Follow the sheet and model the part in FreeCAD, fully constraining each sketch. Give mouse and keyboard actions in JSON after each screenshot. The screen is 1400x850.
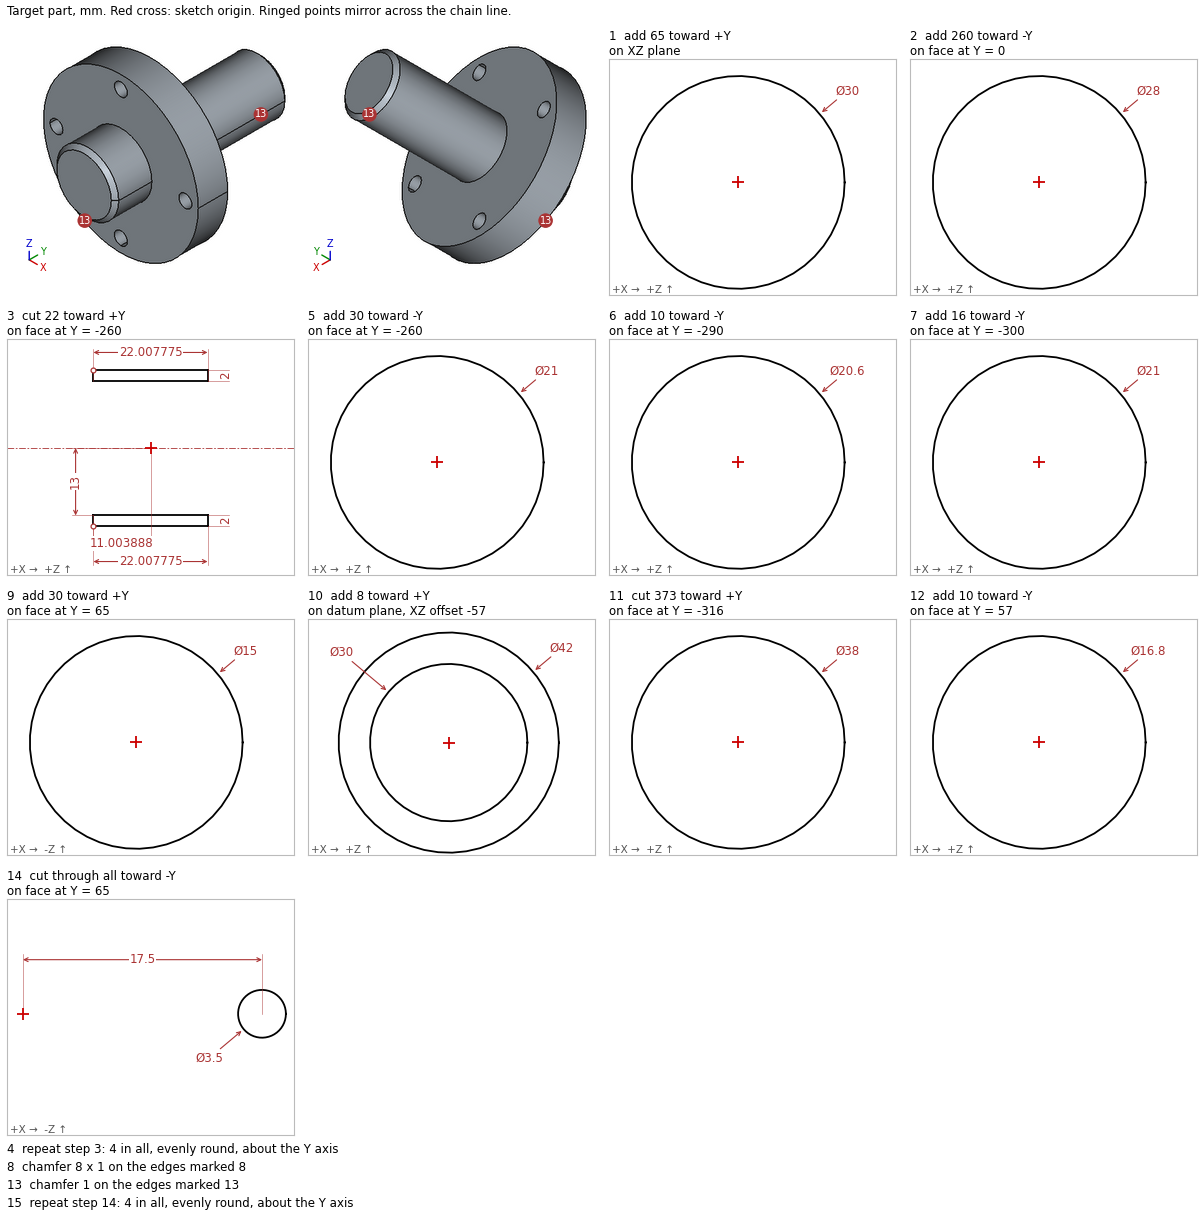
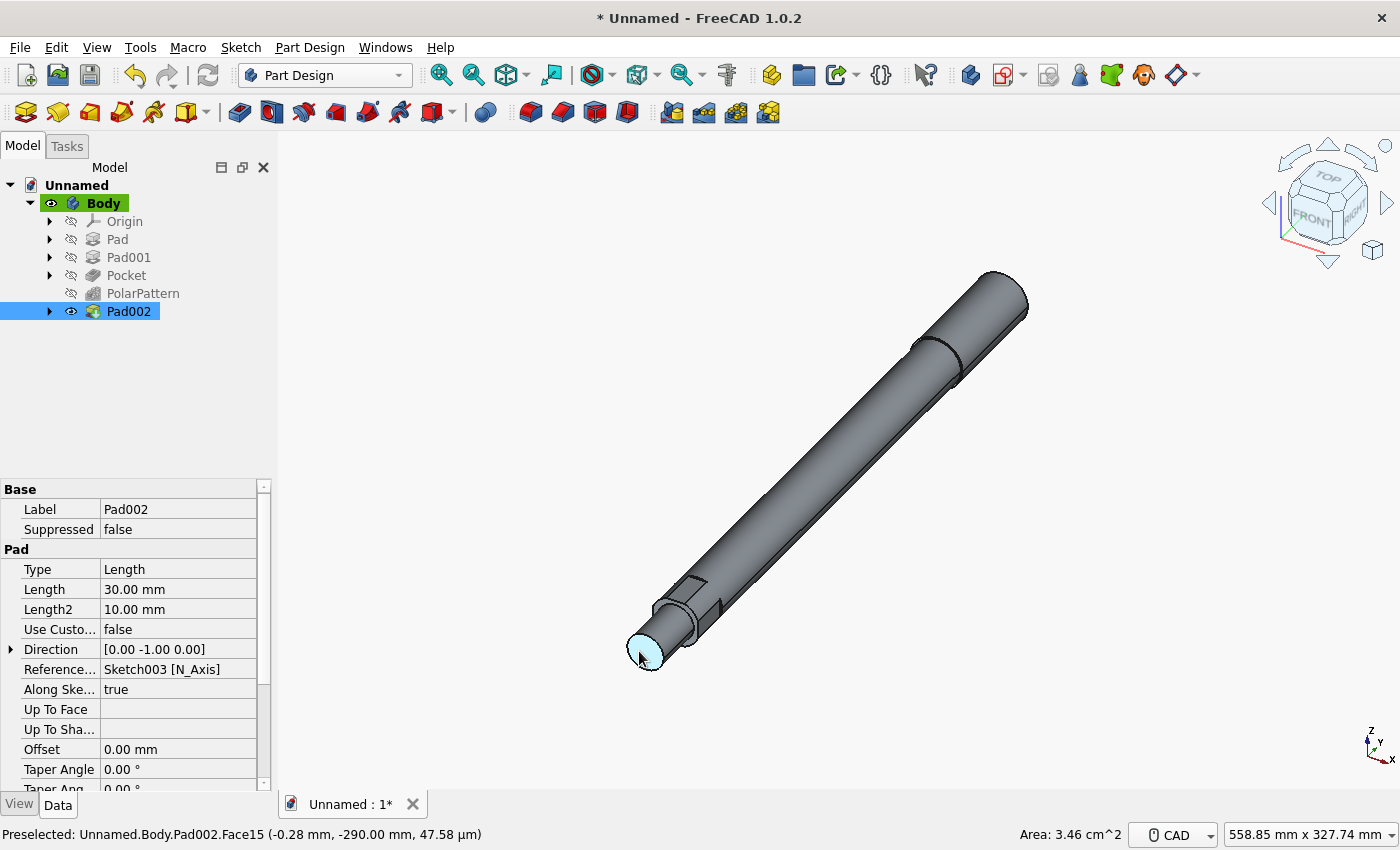
{"action": "left_click", "coordinate": [1004, 76]}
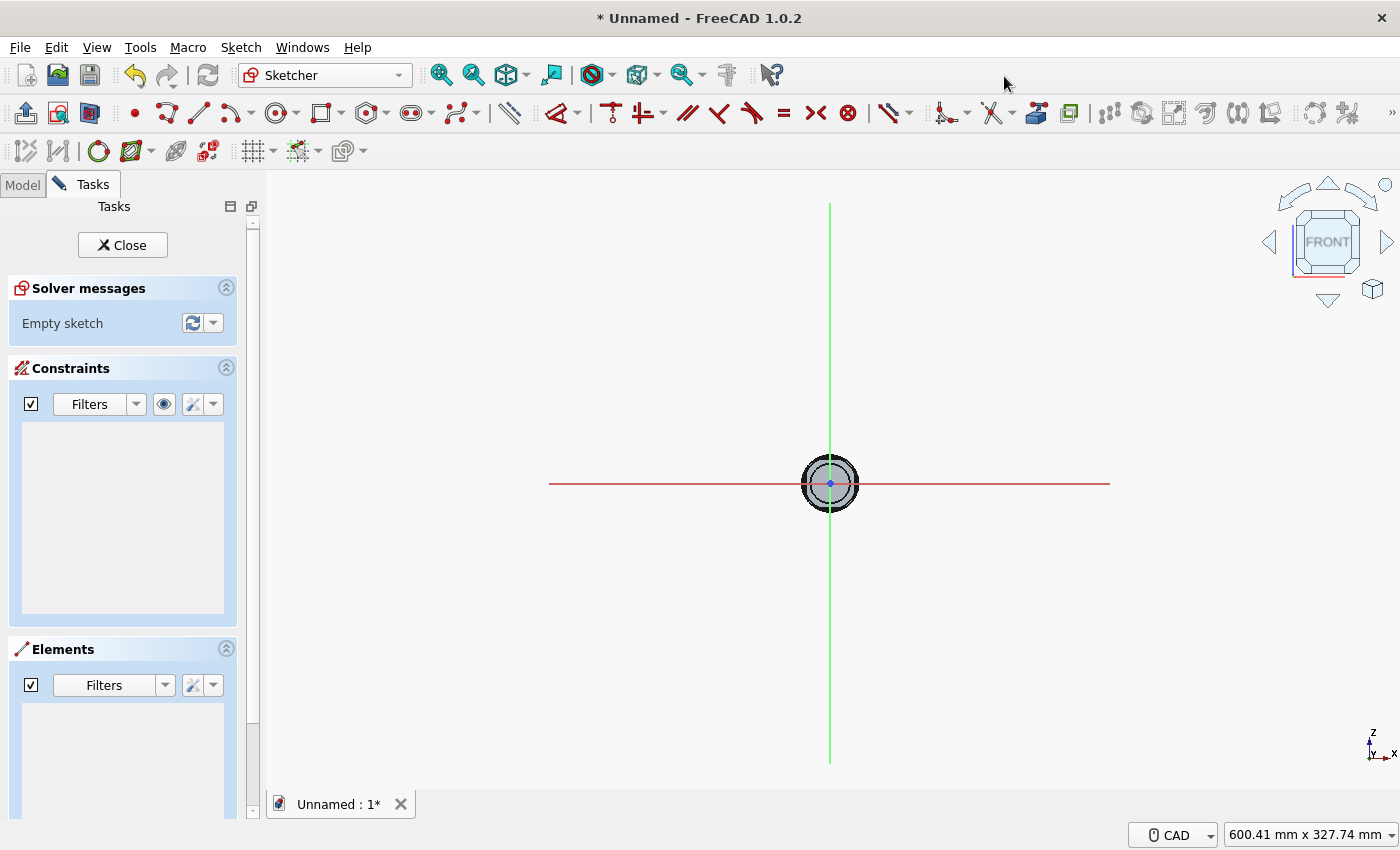
{"action": "scroll", "coordinate": [837, 484], "scroll_direction": "up", "scroll_amount": 12}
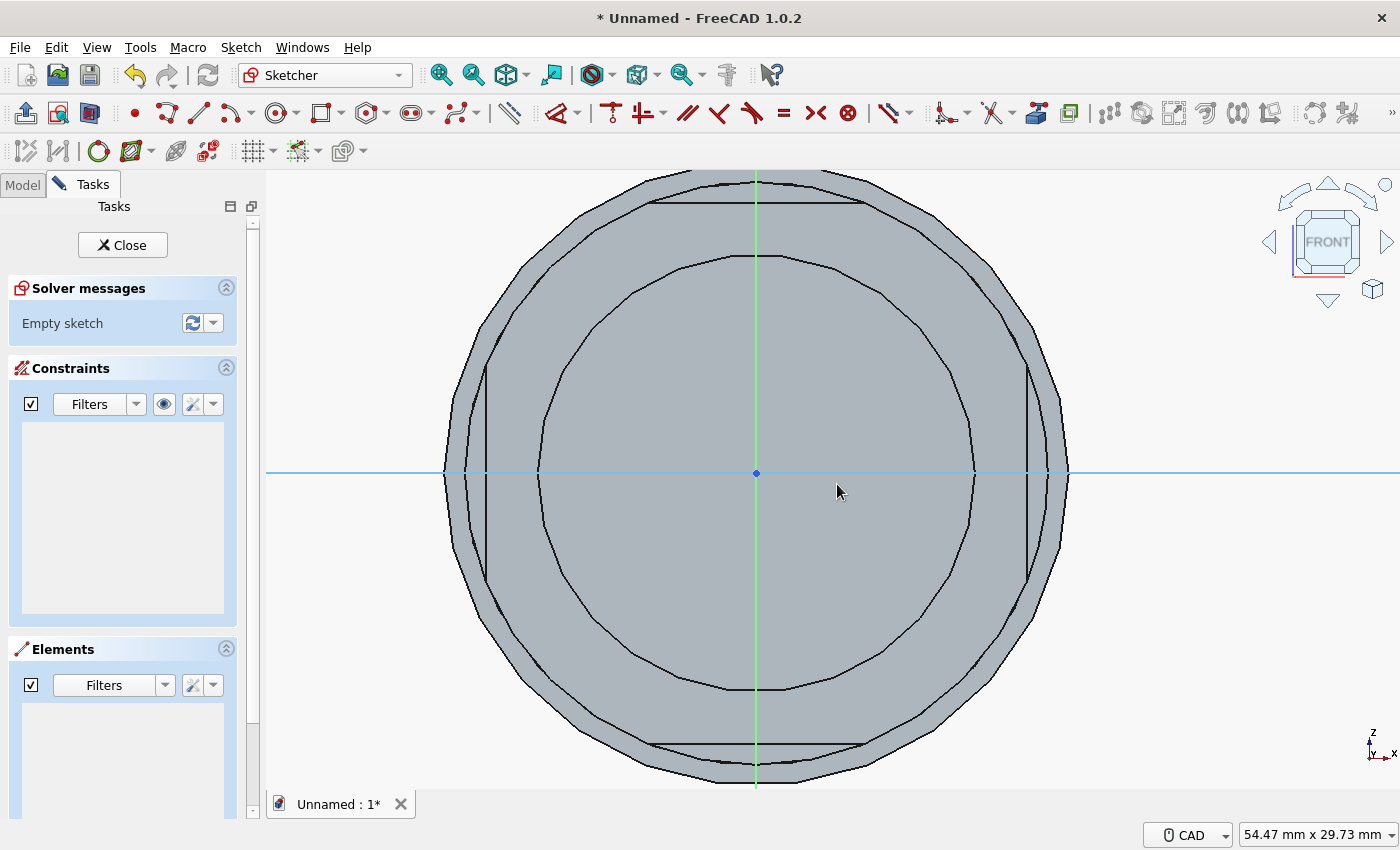
{"action": "left_click", "coordinate": [276, 114]}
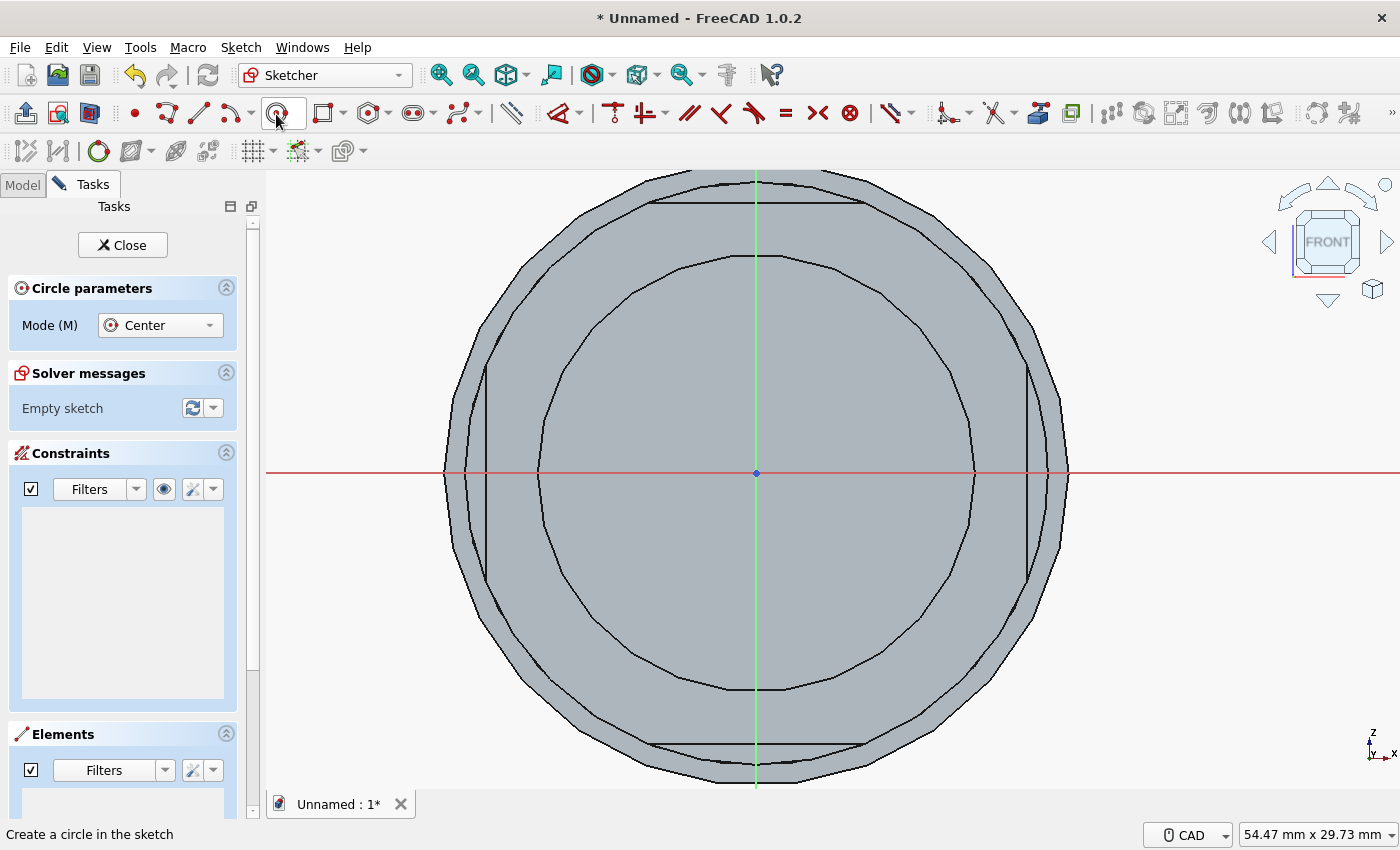
{"action": "left_click", "coordinate": [756, 473]}
{"action": "mouse_move", "coordinate": [908, 322]}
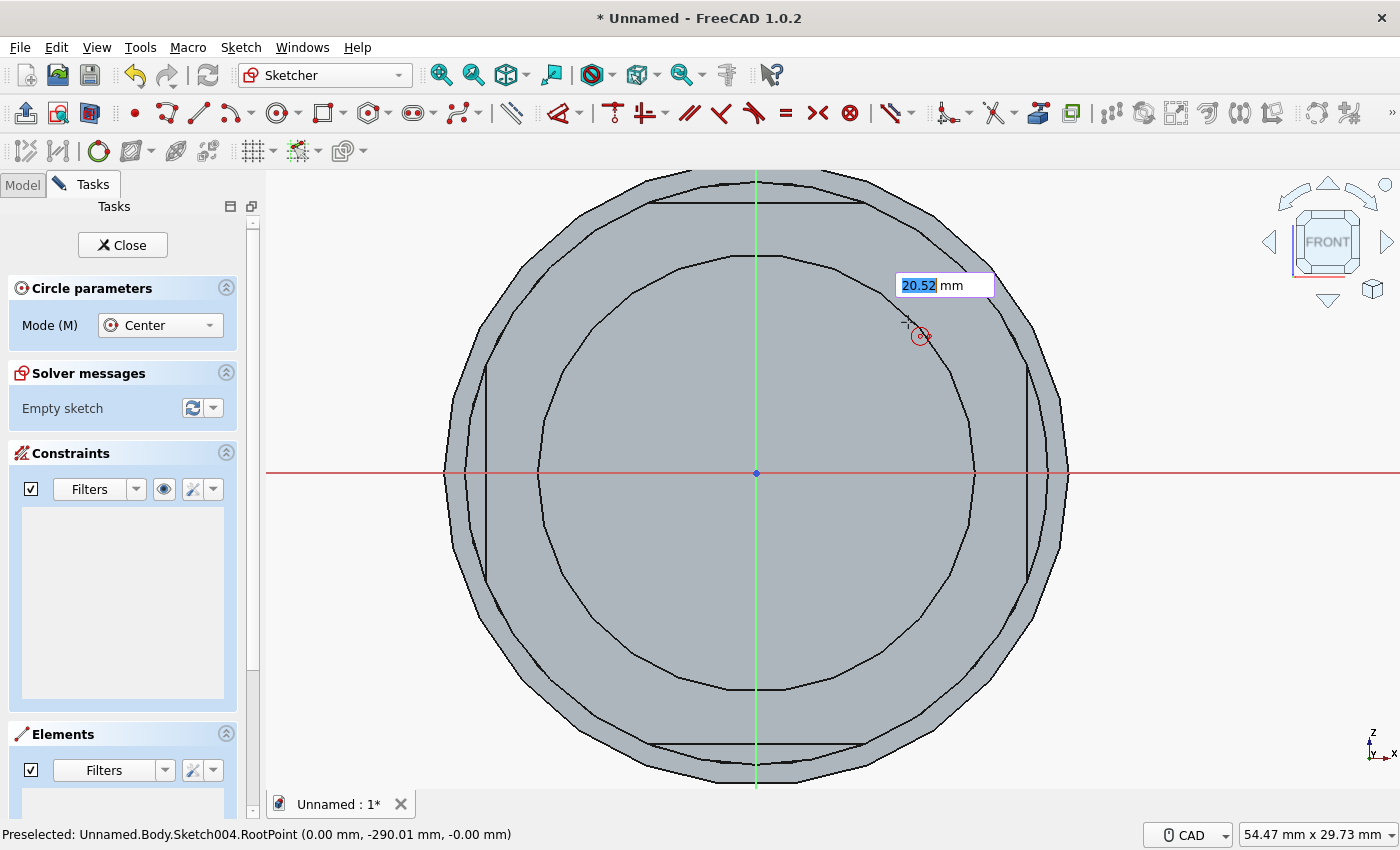
{"action": "type", "text": "20.6"}
{"action": "key", "text": "Return"}
{"action": "key", "text": "Escape"}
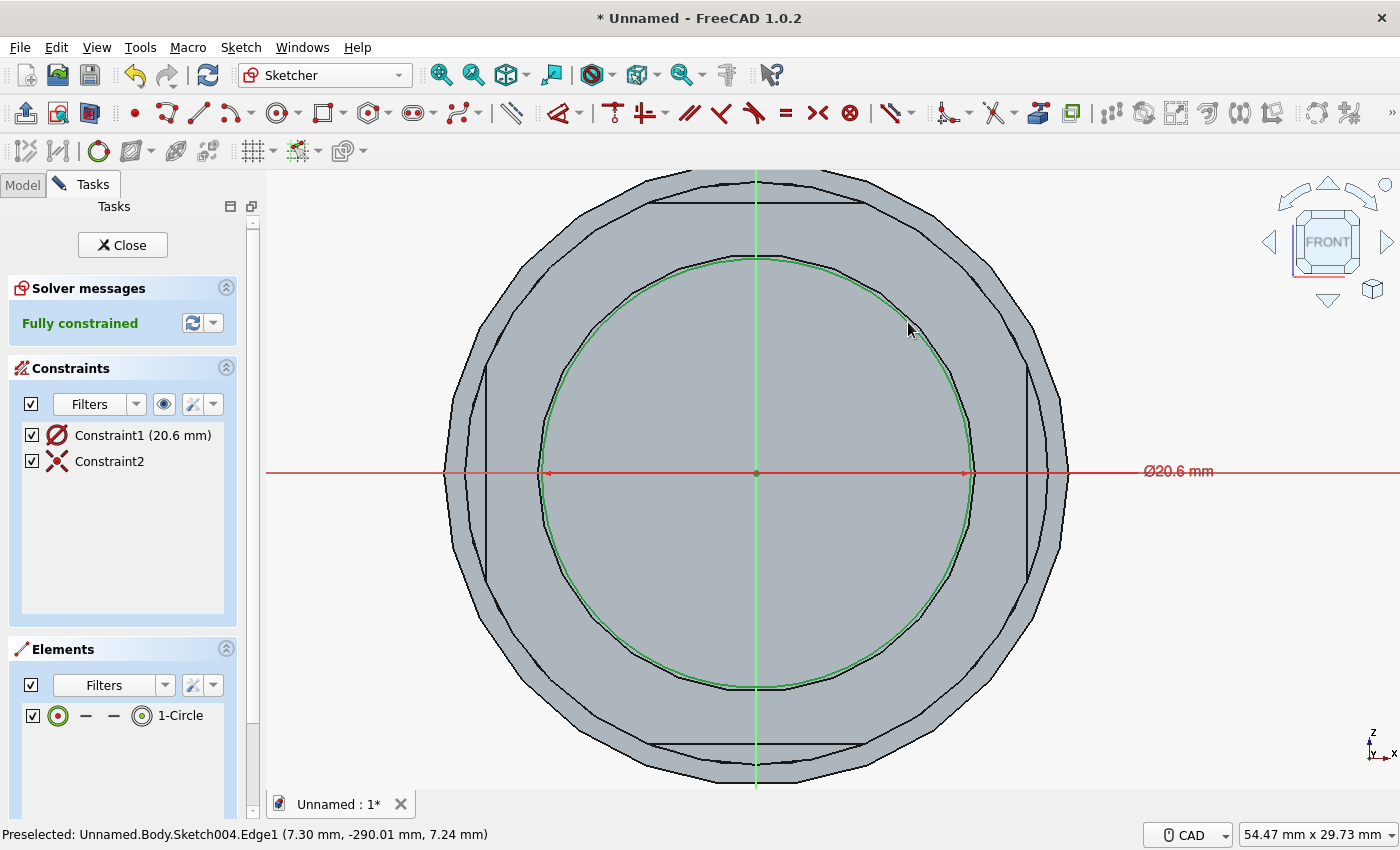
{"action": "left_click", "coordinate": [123, 245]}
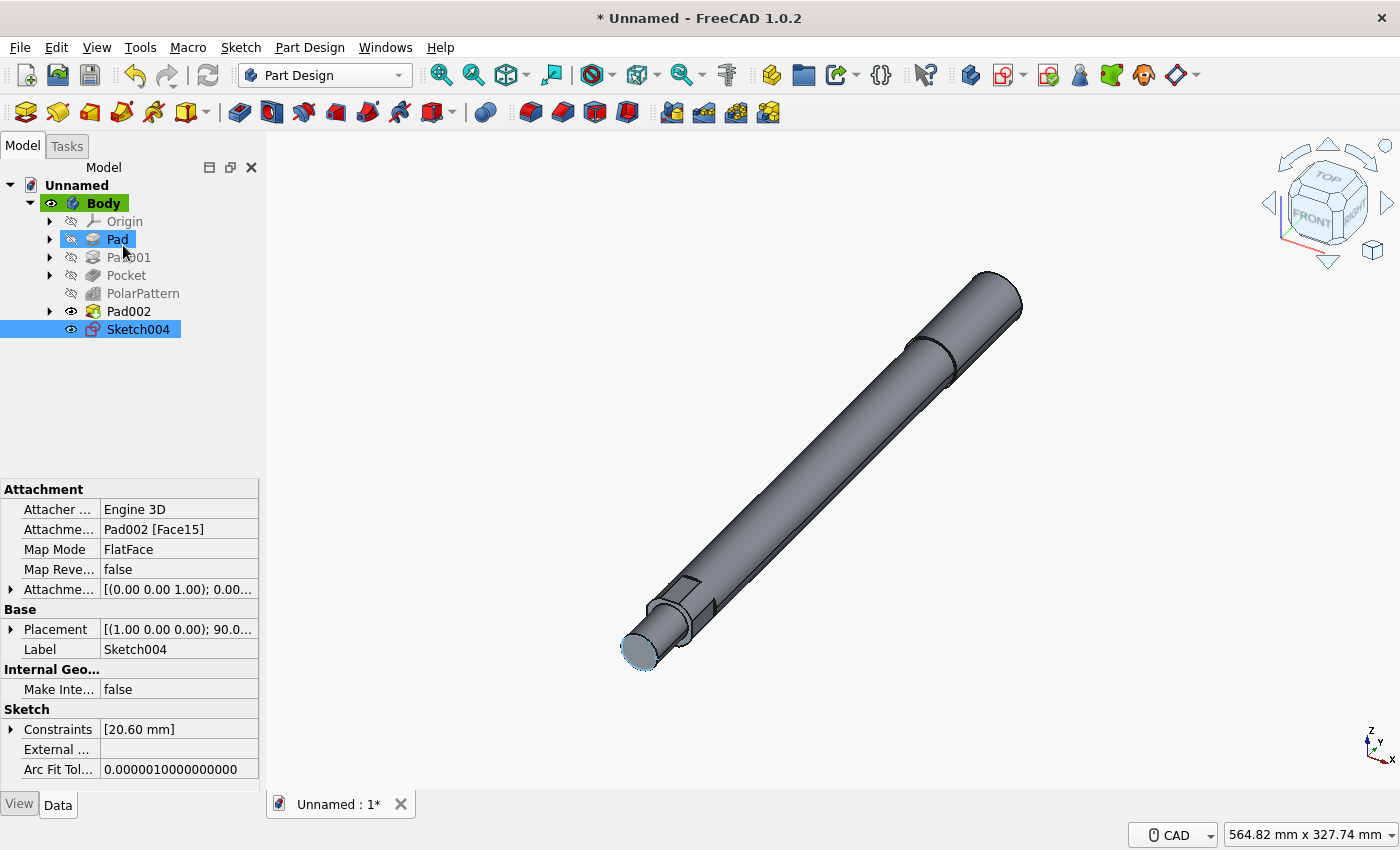
{"action": "left_click", "coordinate": [26, 112]}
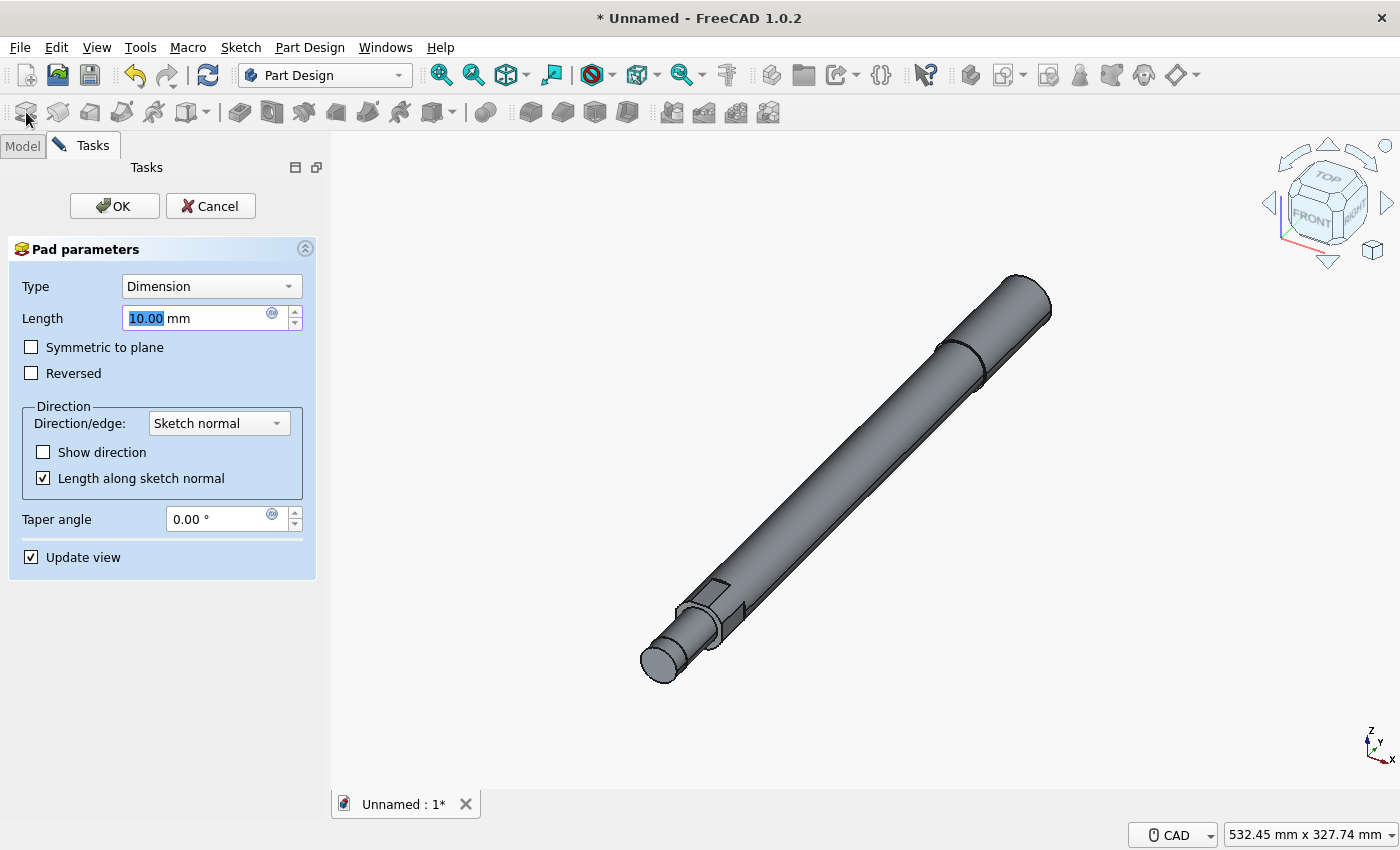
{"action": "type", "text": "10"}
{"action": "key", "text": "Tab"}